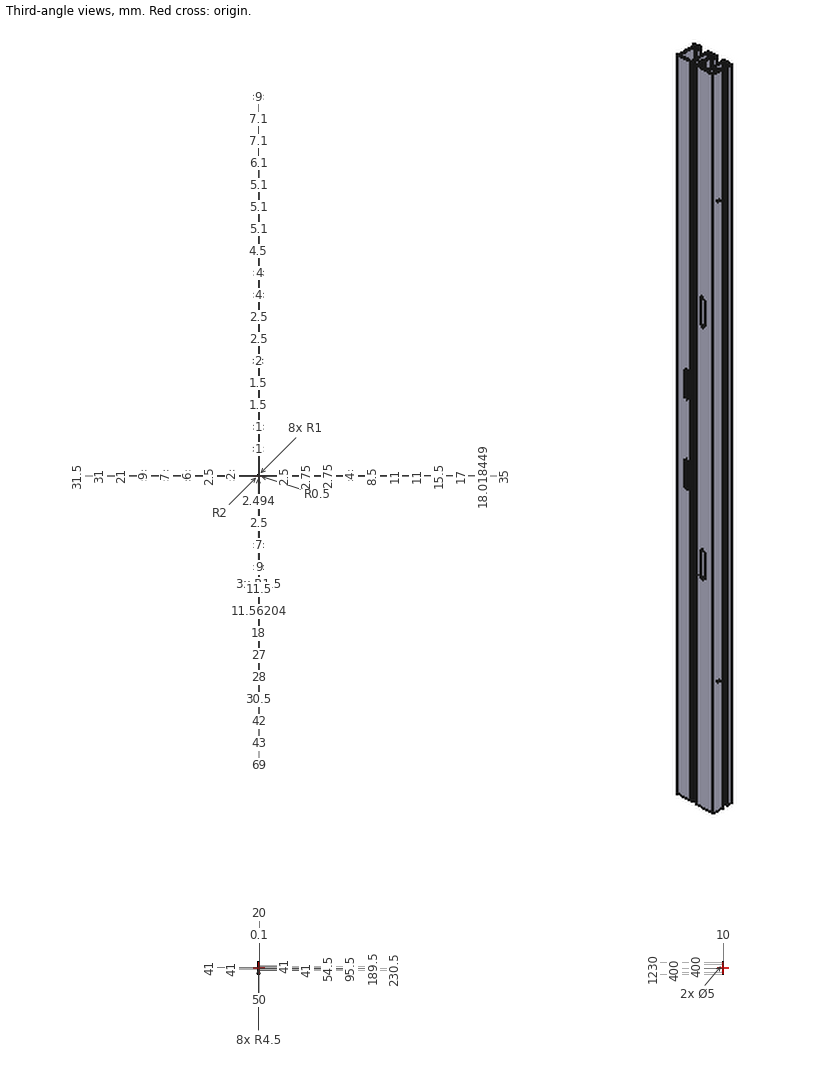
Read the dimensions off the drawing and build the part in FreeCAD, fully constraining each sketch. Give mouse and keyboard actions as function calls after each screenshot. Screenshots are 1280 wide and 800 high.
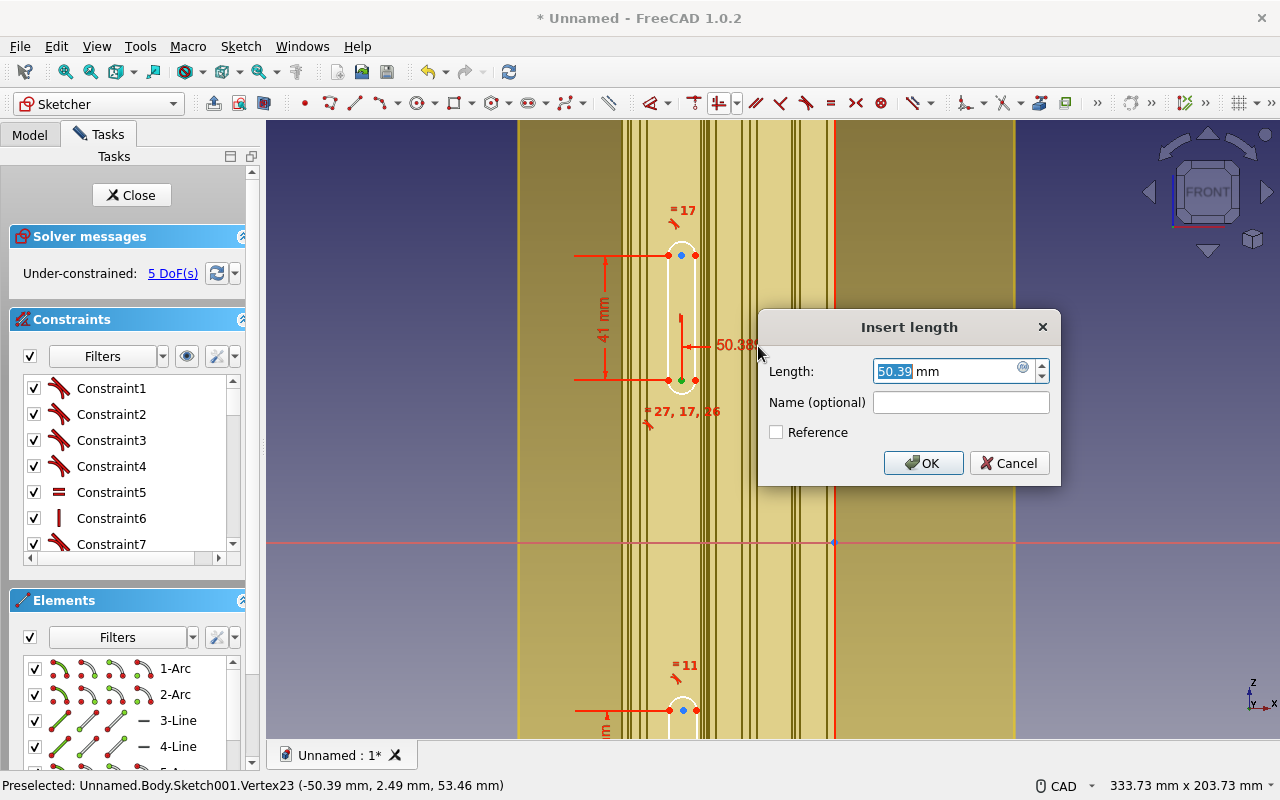
text(50)
key(Return)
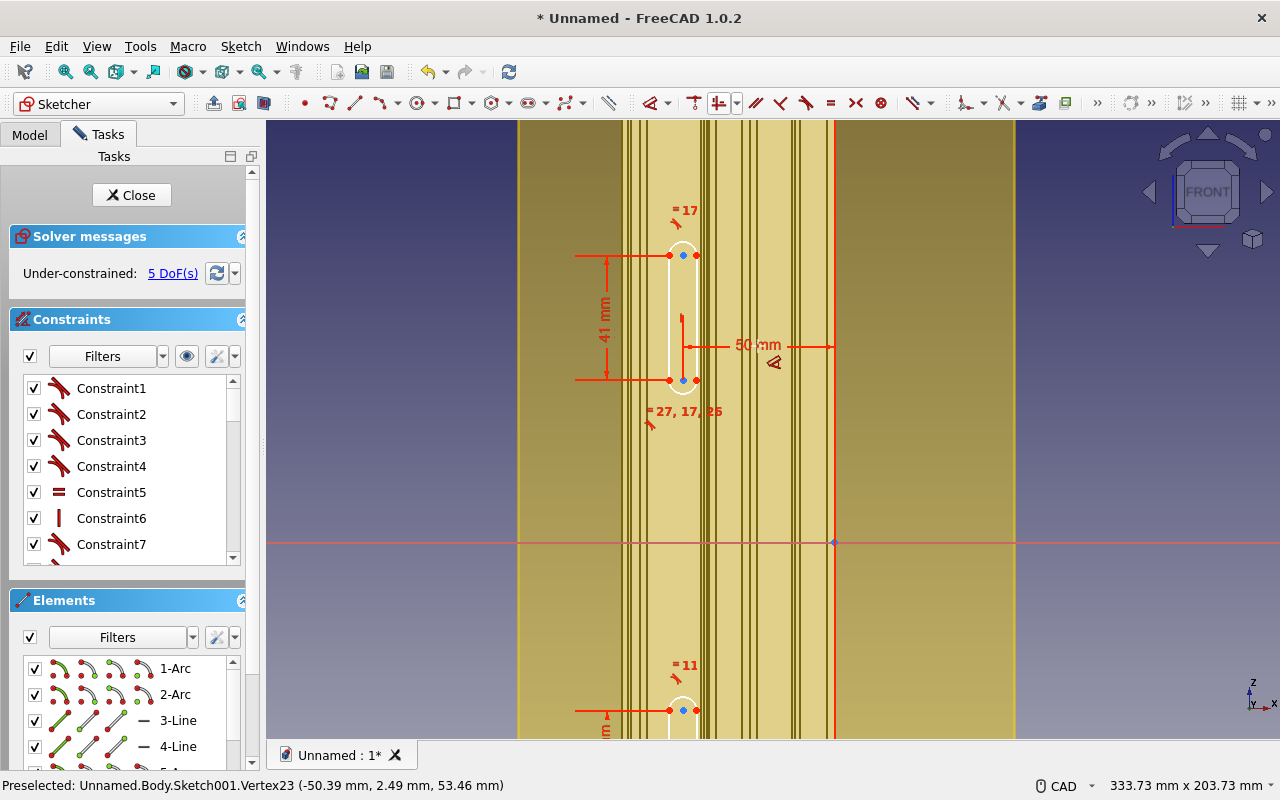
scroll(684, 381, down, 6)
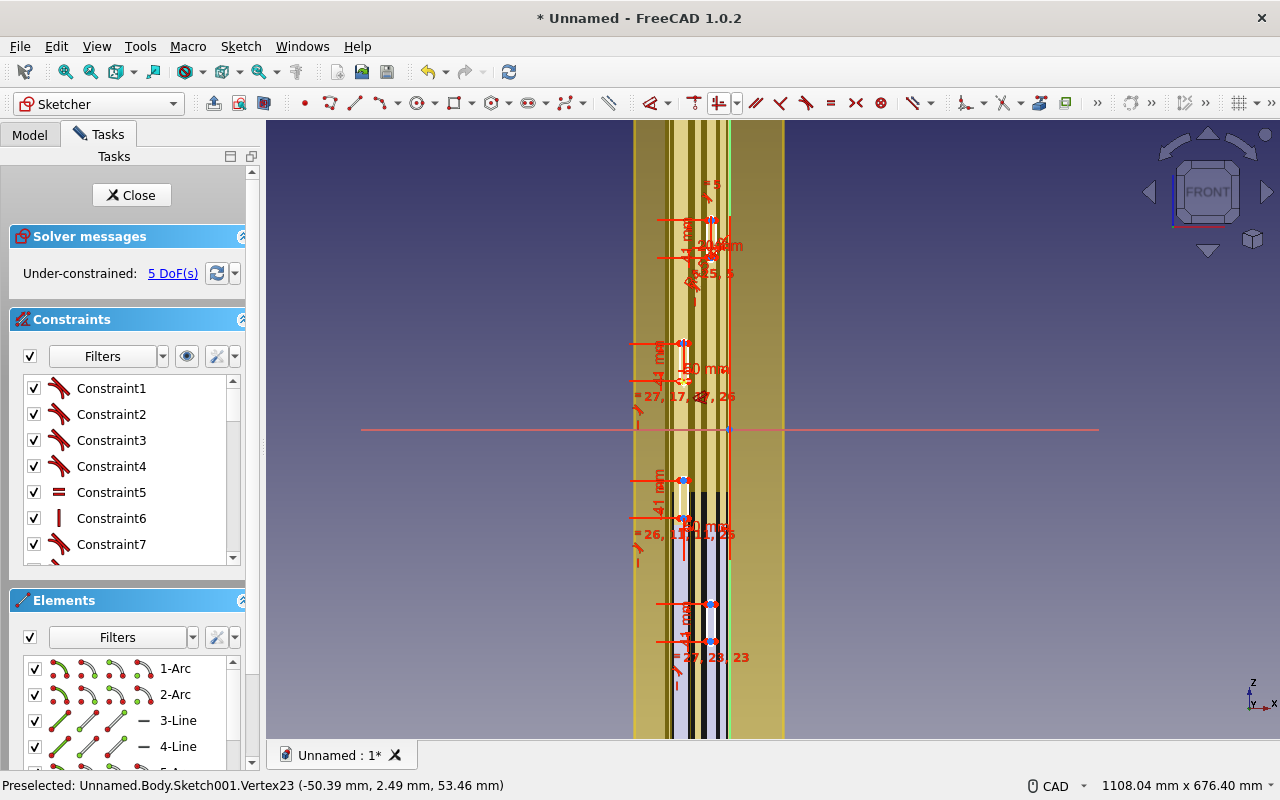
scroll(711, 642, up, 6)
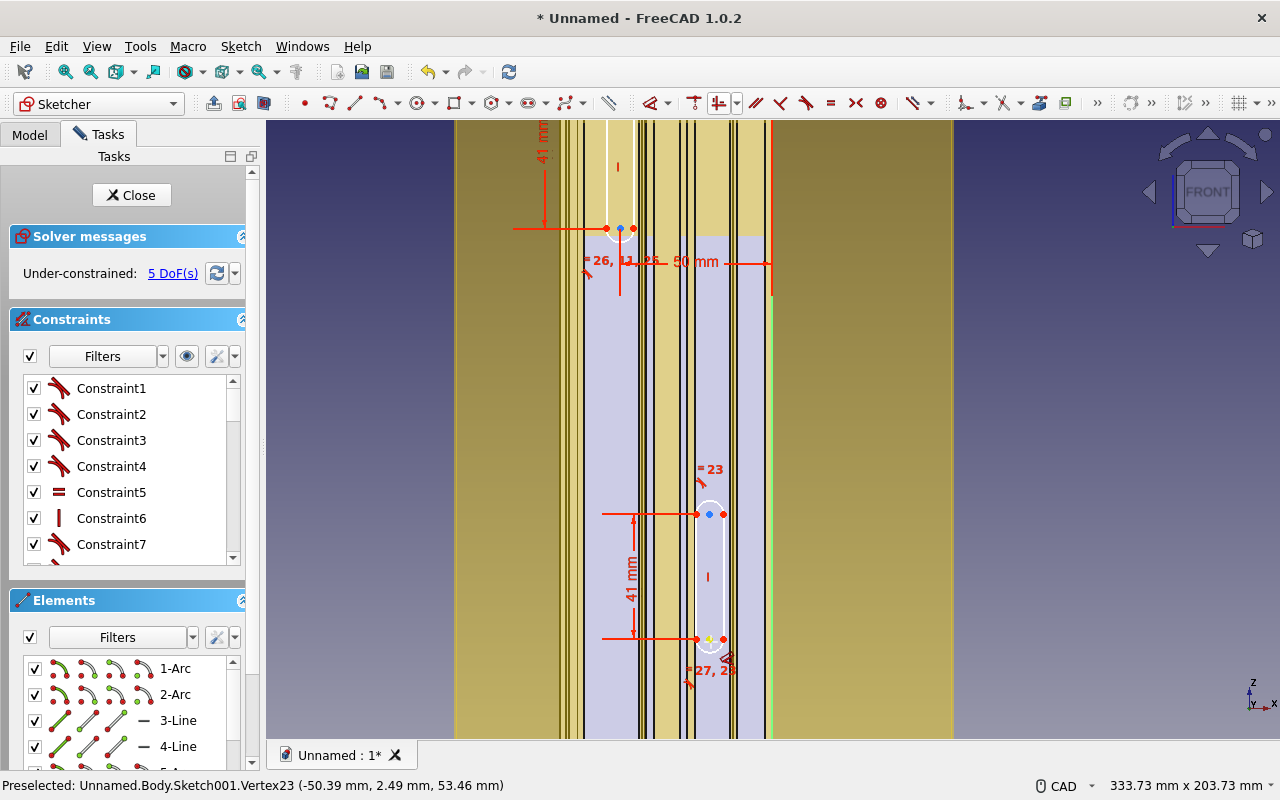
click(710, 639)
click(741, 673)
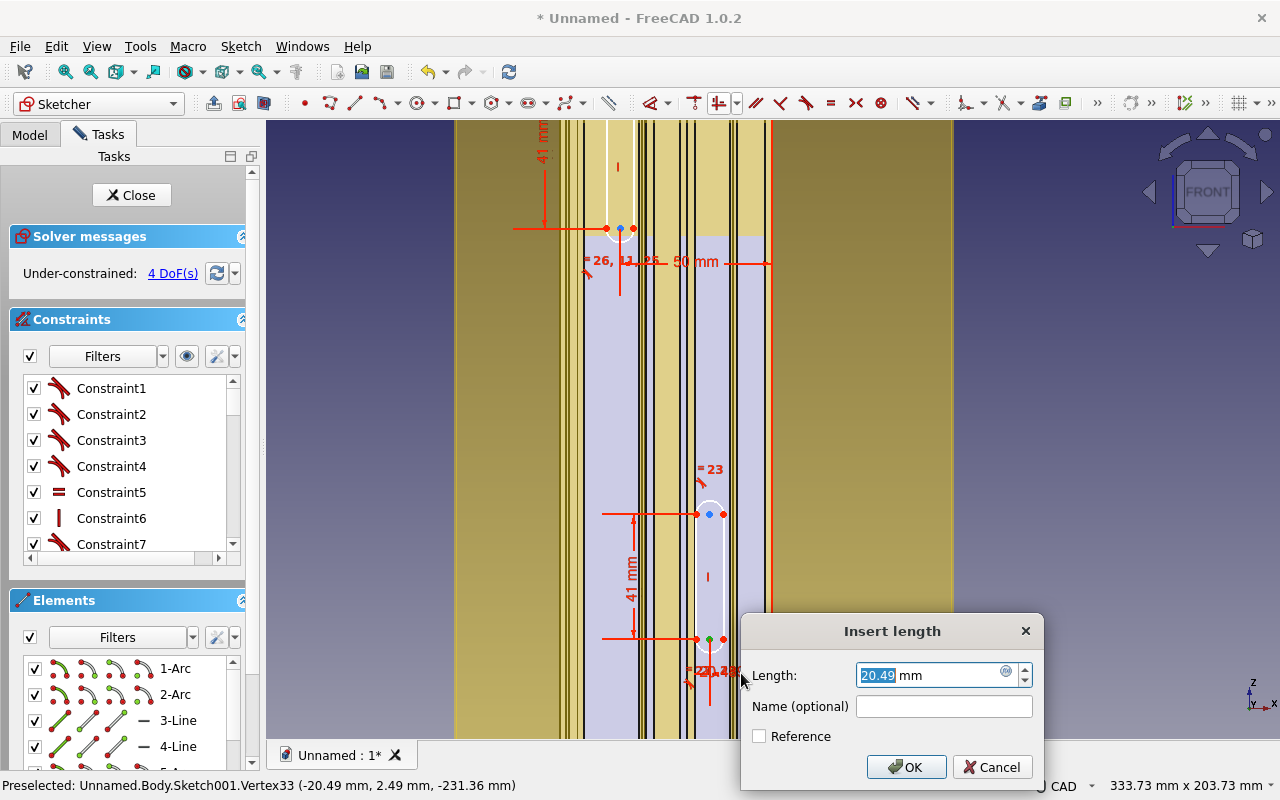
text(20)
key(Return)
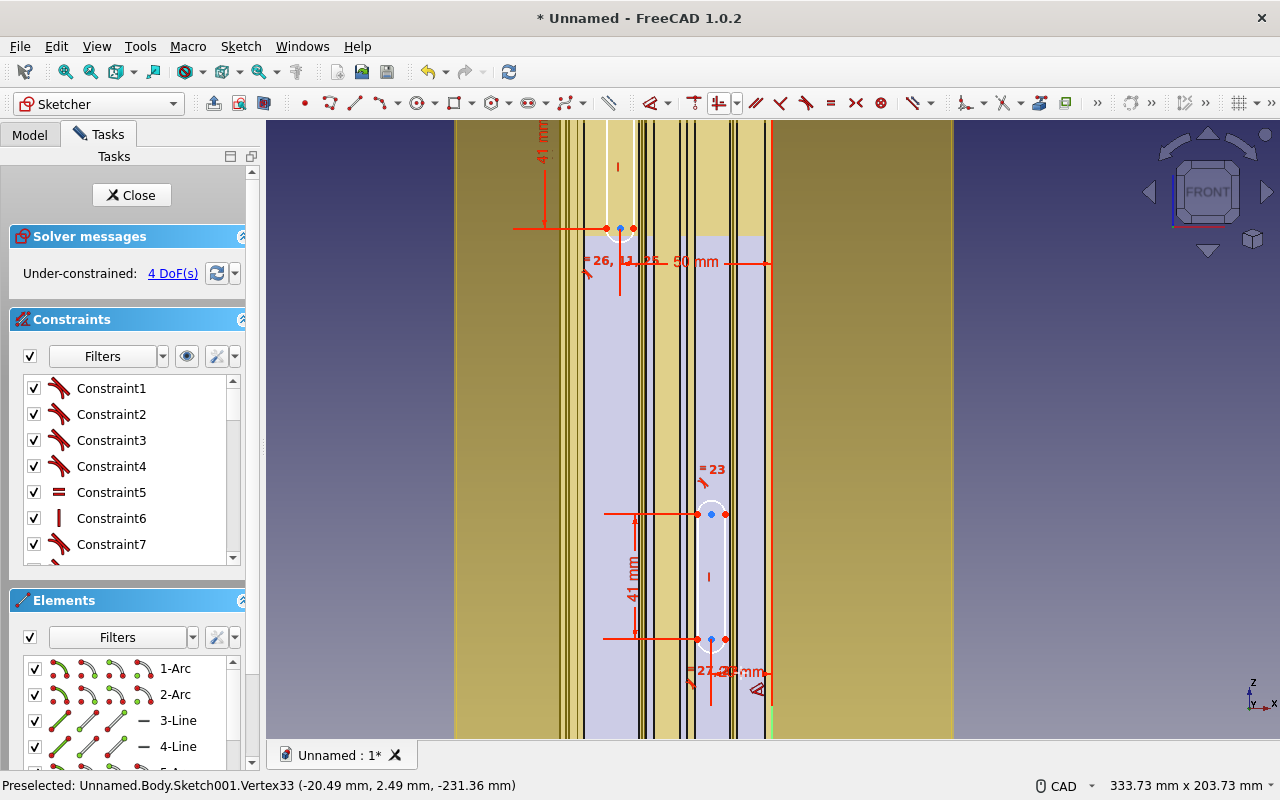
click(607, 229)
click(573, 188)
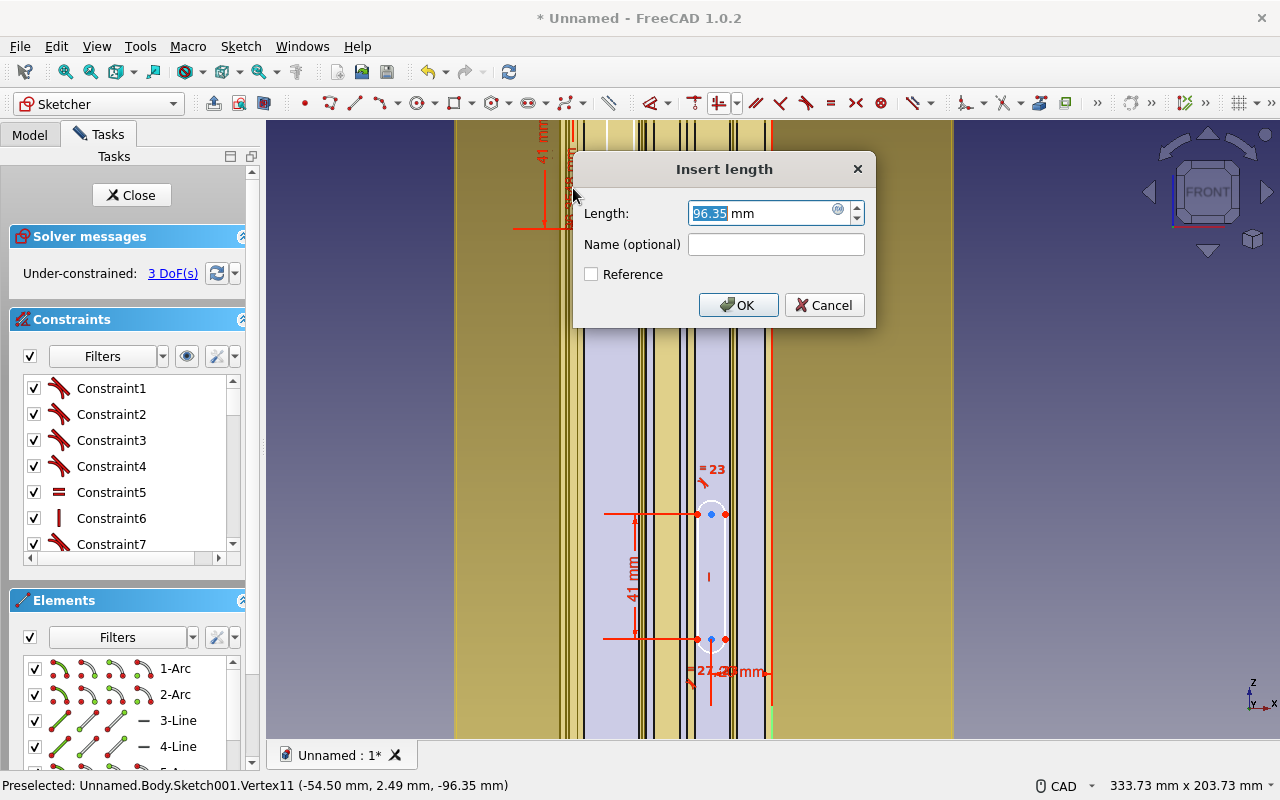
text(95.5)
key(Return)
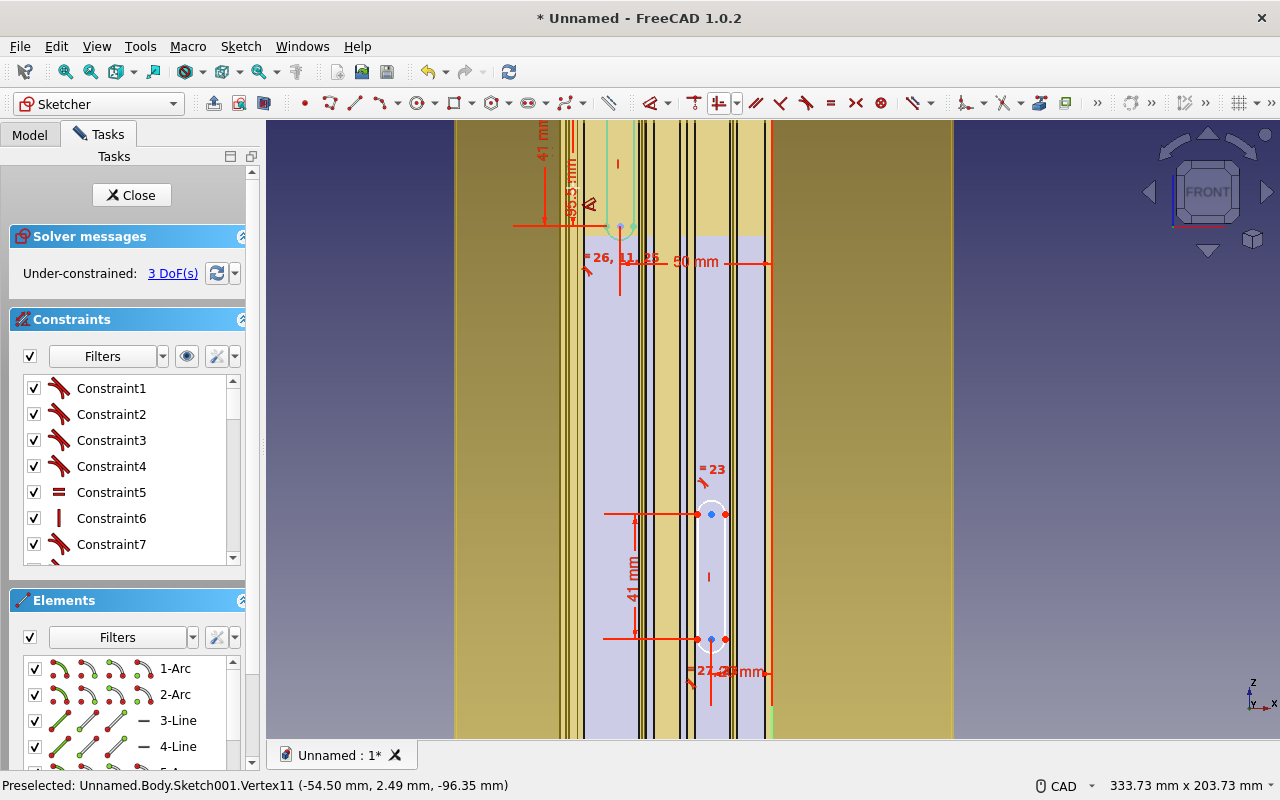
scroll(711, 642, down, 6)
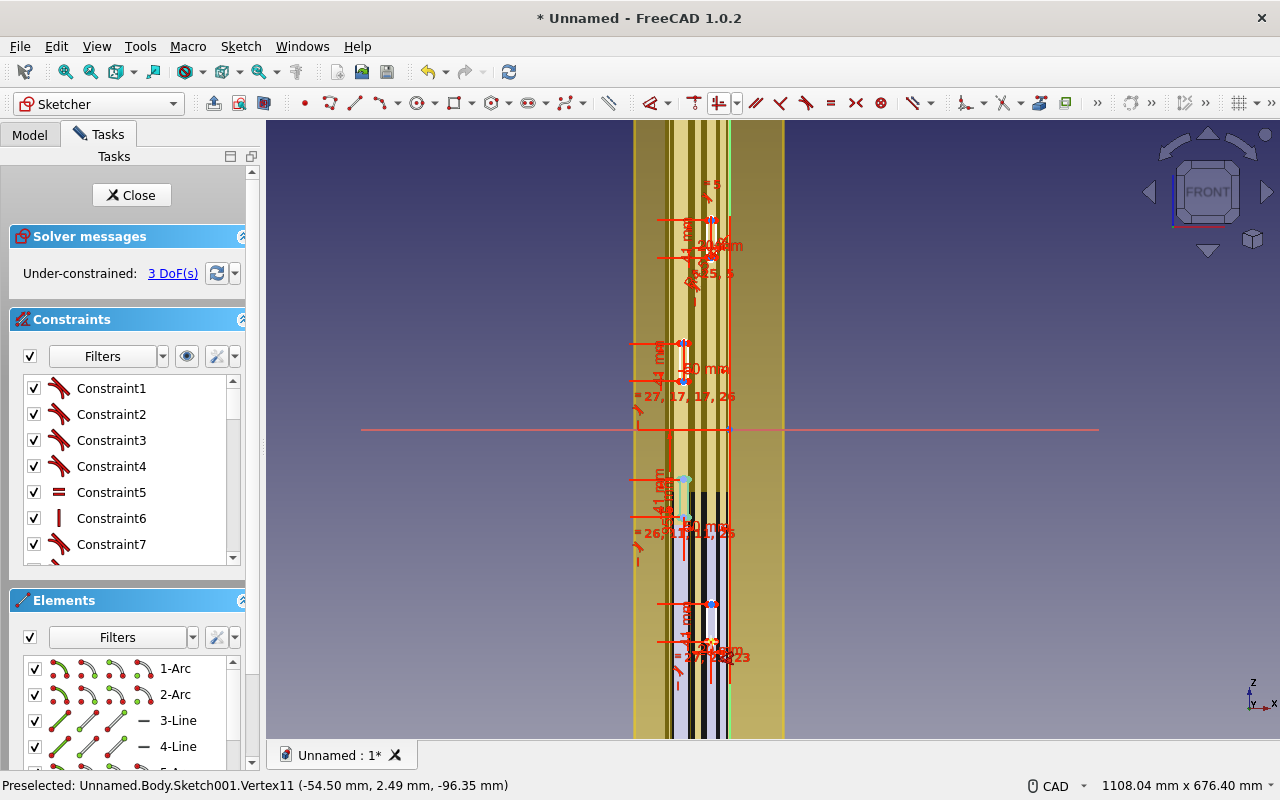
scroll(680, 381, up, 6)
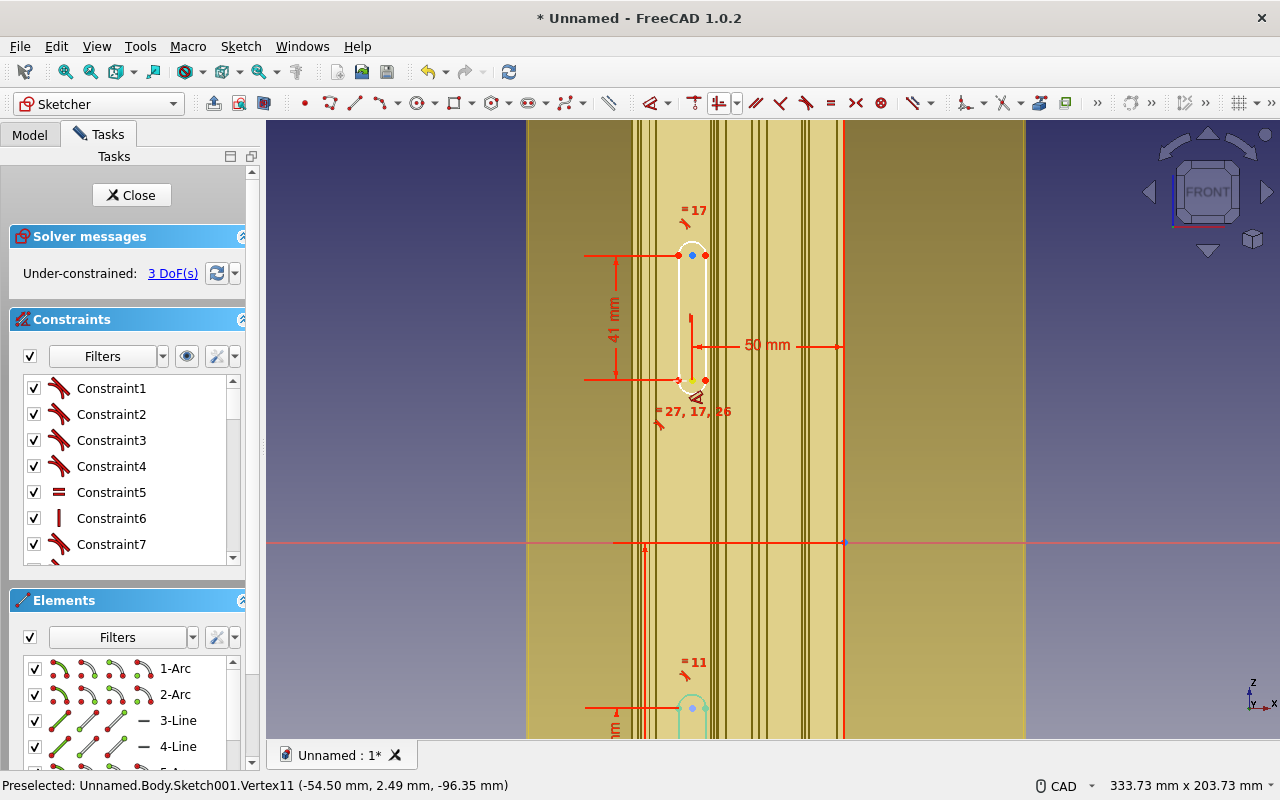
click(679, 380)
click(878, 461)